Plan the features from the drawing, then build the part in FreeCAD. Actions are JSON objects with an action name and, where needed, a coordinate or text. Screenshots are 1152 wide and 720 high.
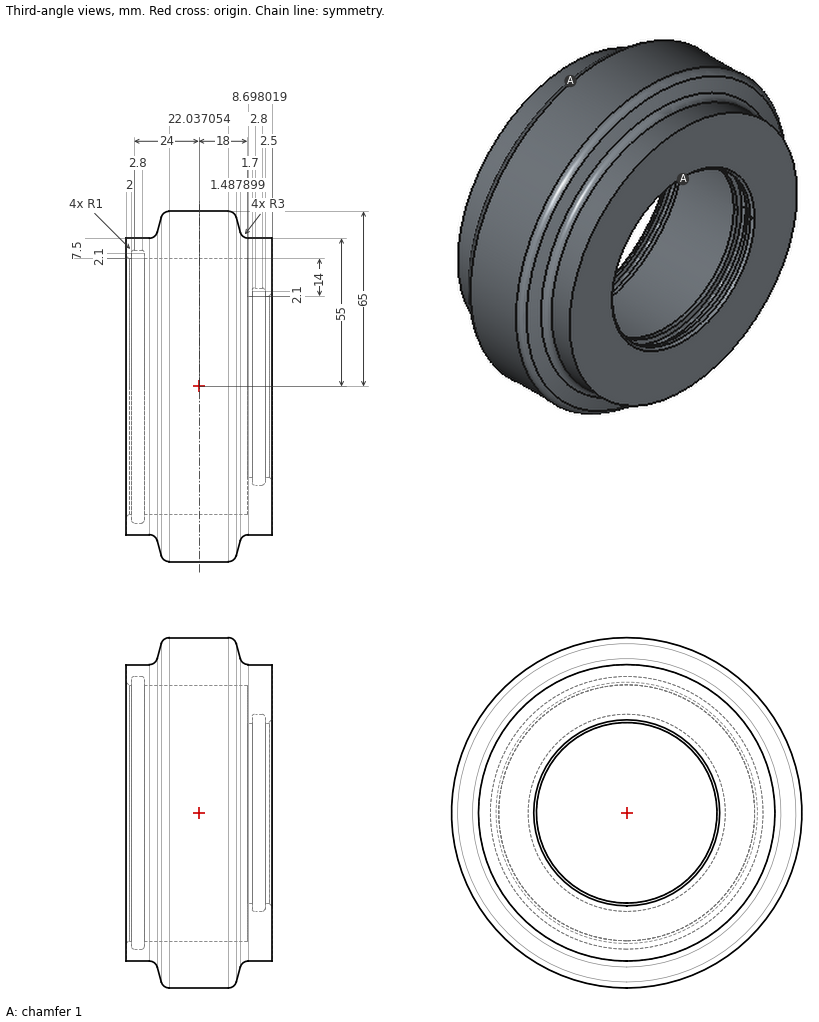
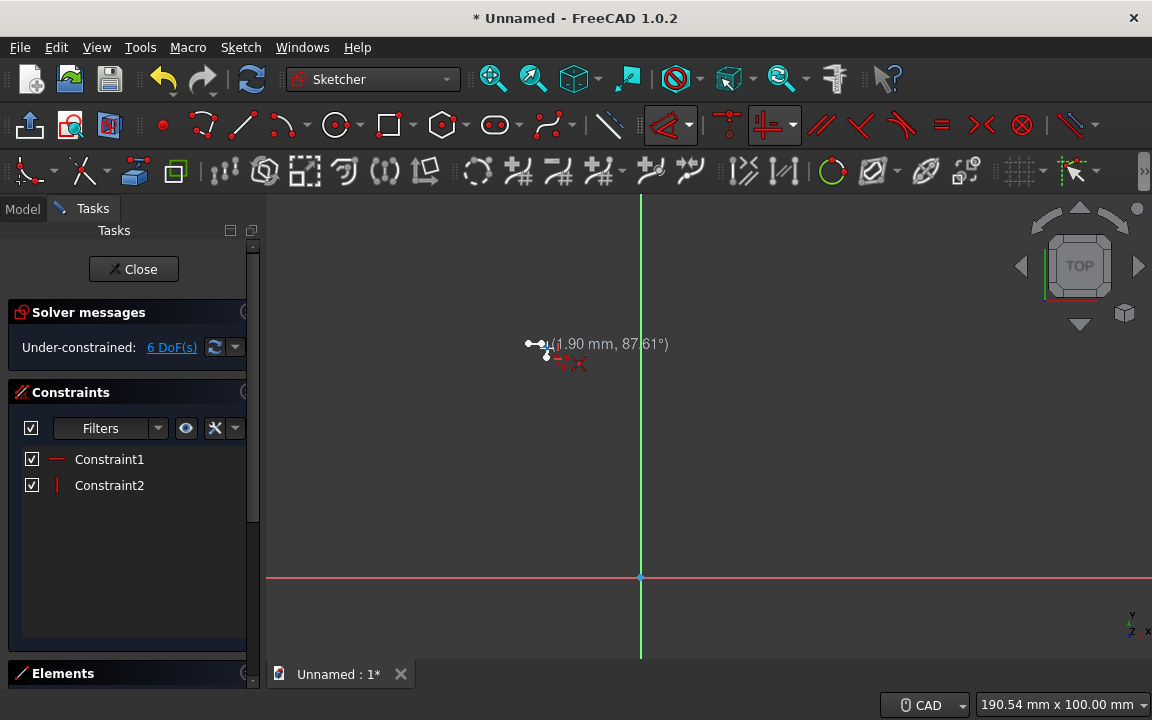
{"action": "left_click", "coordinate": [724, 357]}
{"action": "left_click", "coordinate": [724, 422]}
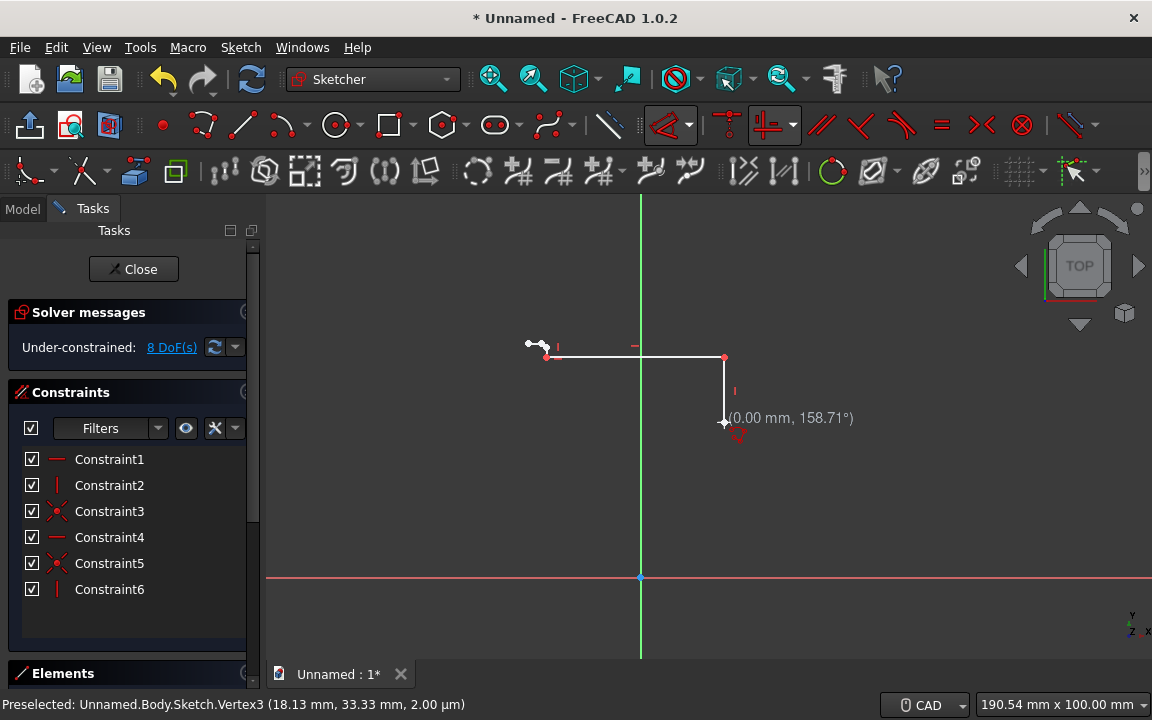
{"action": "scroll", "coordinate": [732, 422], "scroll_direction": "up", "scroll_amount": 4}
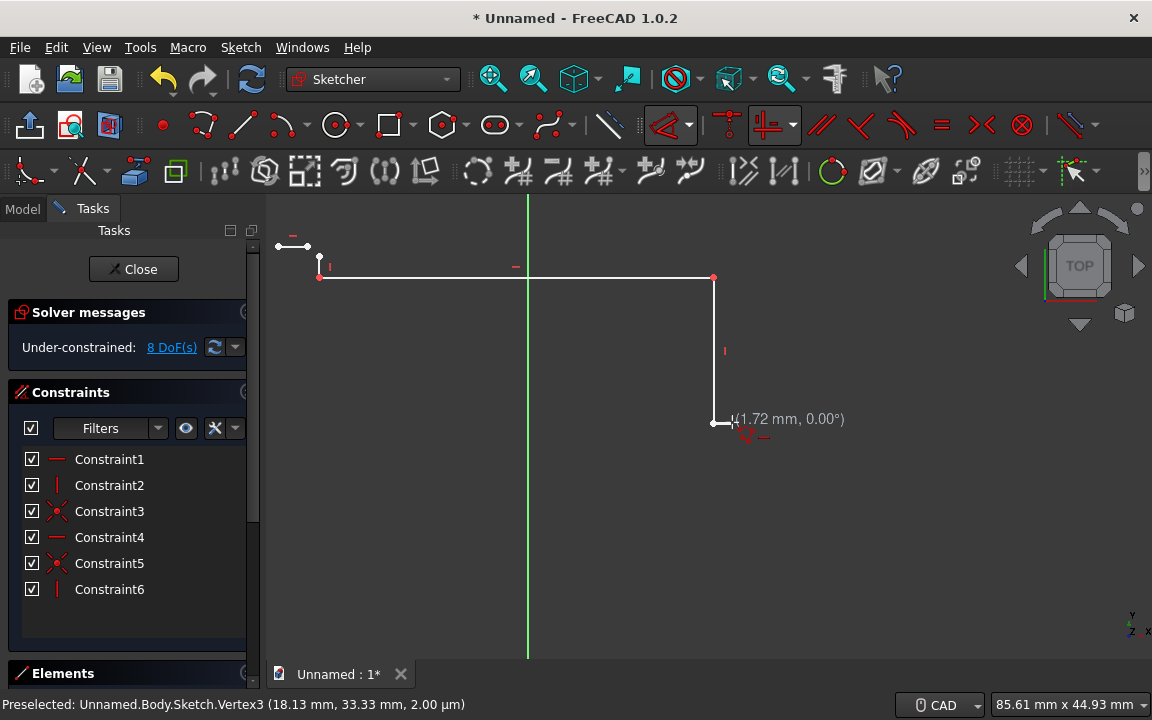
{"action": "left_click", "coordinate": [732, 421]}
{"action": "left_click", "coordinate": [732, 400]}
{"action": "right_click", "coordinate": [732, 400]}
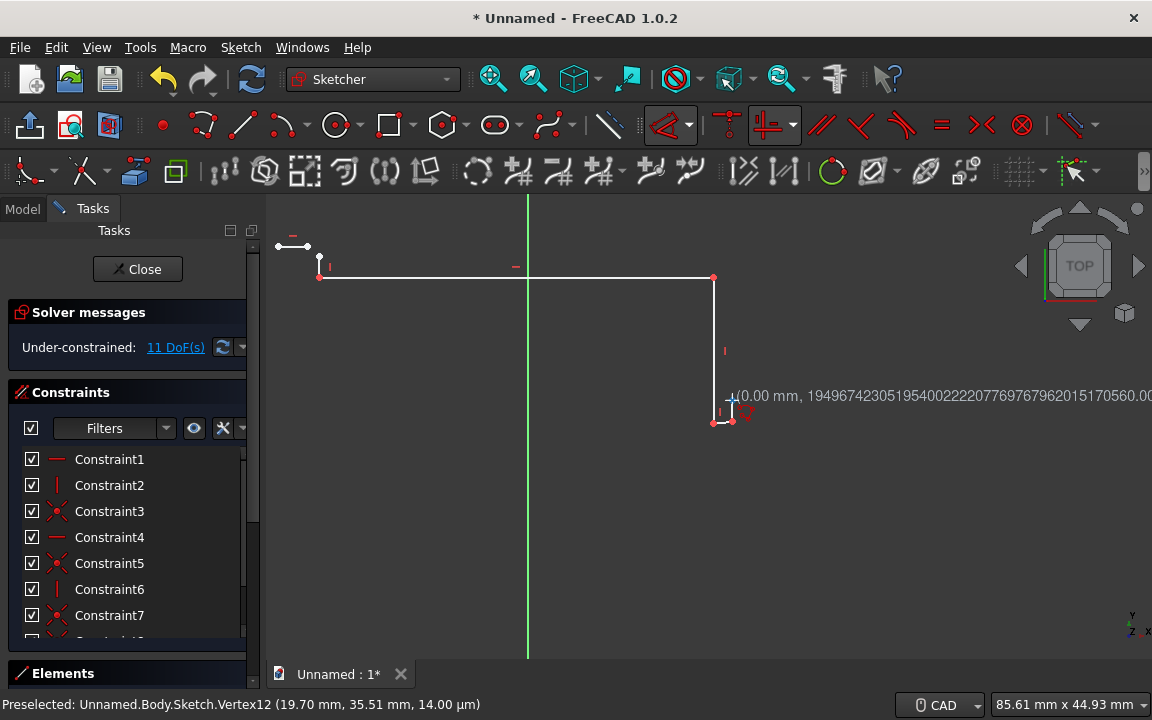
{"action": "key", "text": "g l"}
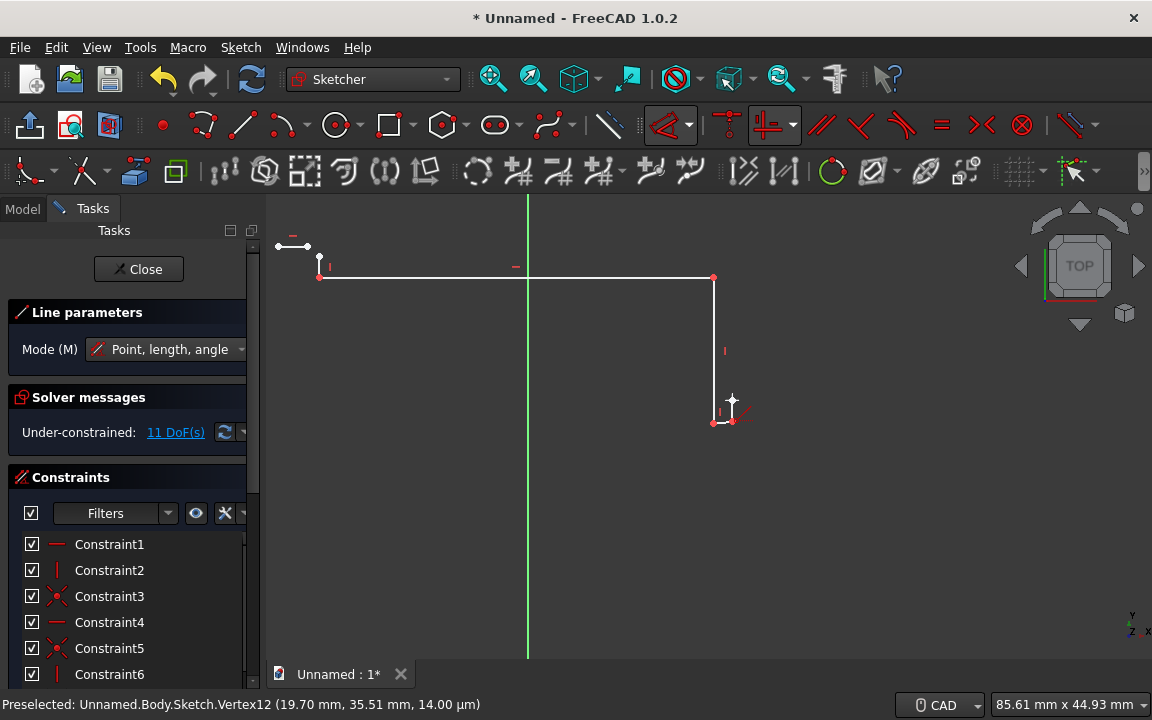
{"action": "left_click", "coordinate": [742, 390]}
{"action": "left_click", "coordinate": [771, 390]}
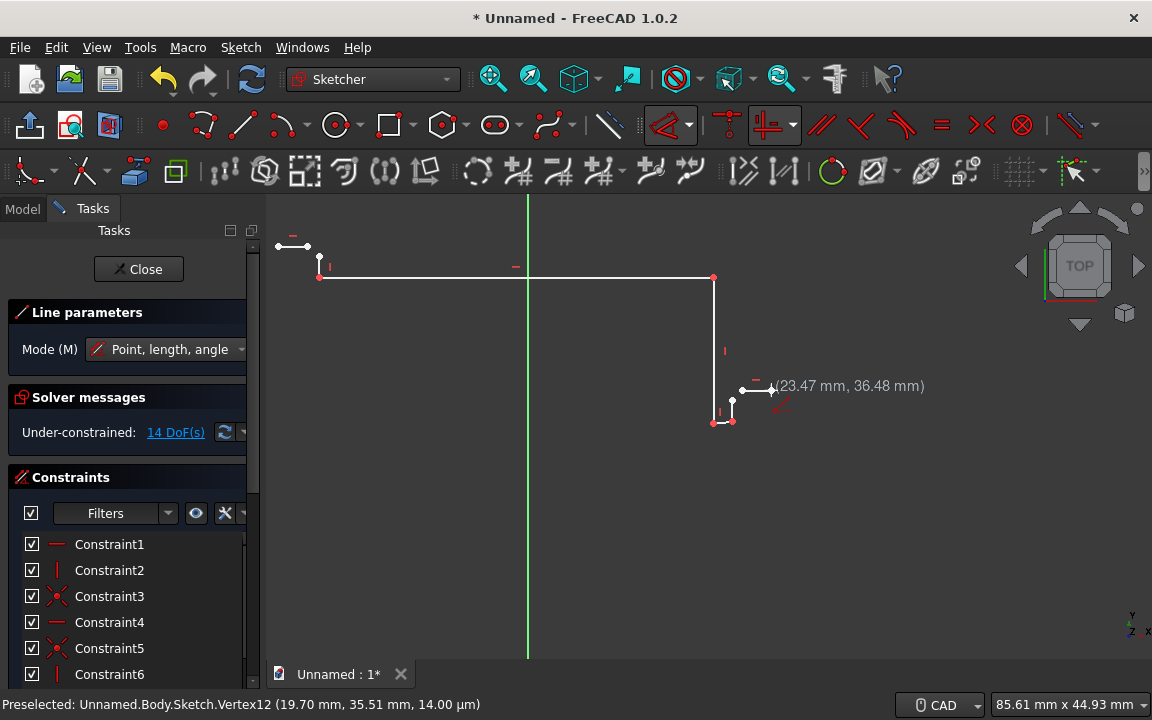
{"action": "left_click", "coordinate": [204, 126]}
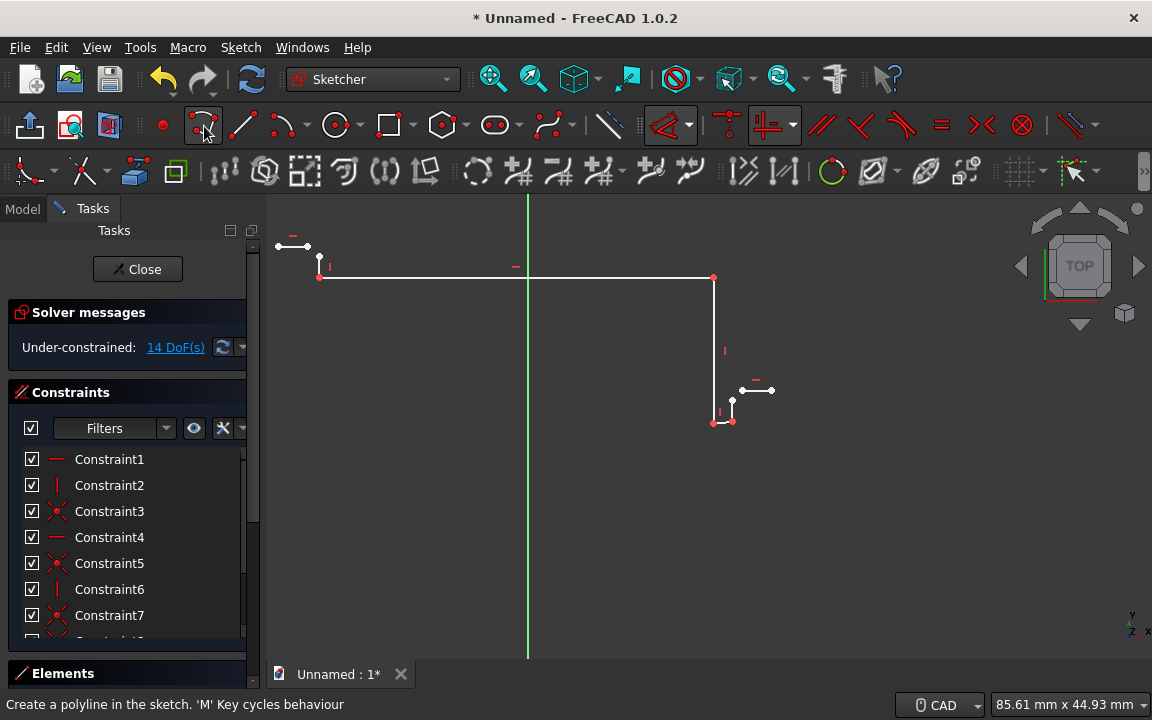
{"action": "left_click", "coordinate": [782, 400]}
{"action": "left_click", "coordinate": [782, 422]}
{"action": "left_click", "coordinate": [808, 422]}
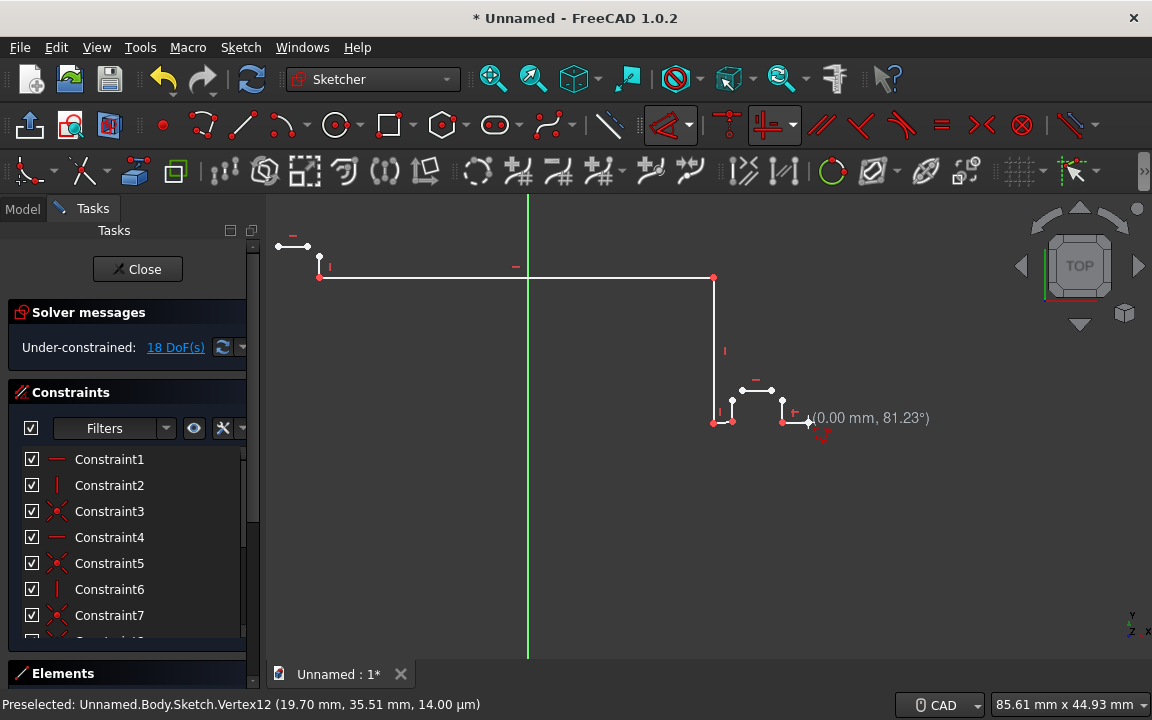
{"action": "scroll", "coordinate": [732, 422], "scroll_direction": "down", "scroll_amount": 4}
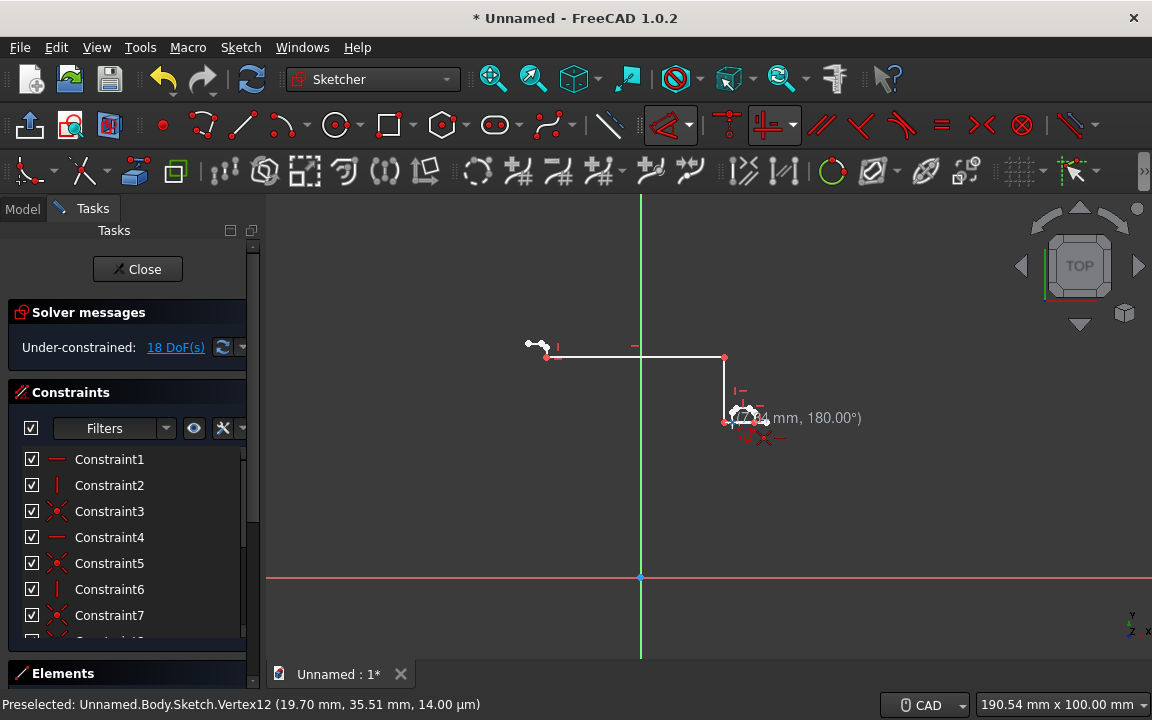
{"action": "left_click", "coordinate": [766, 322]}
{"action": "left_click", "coordinate": [726, 322]}
{"action": "right_click", "coordinate": [726, 322]}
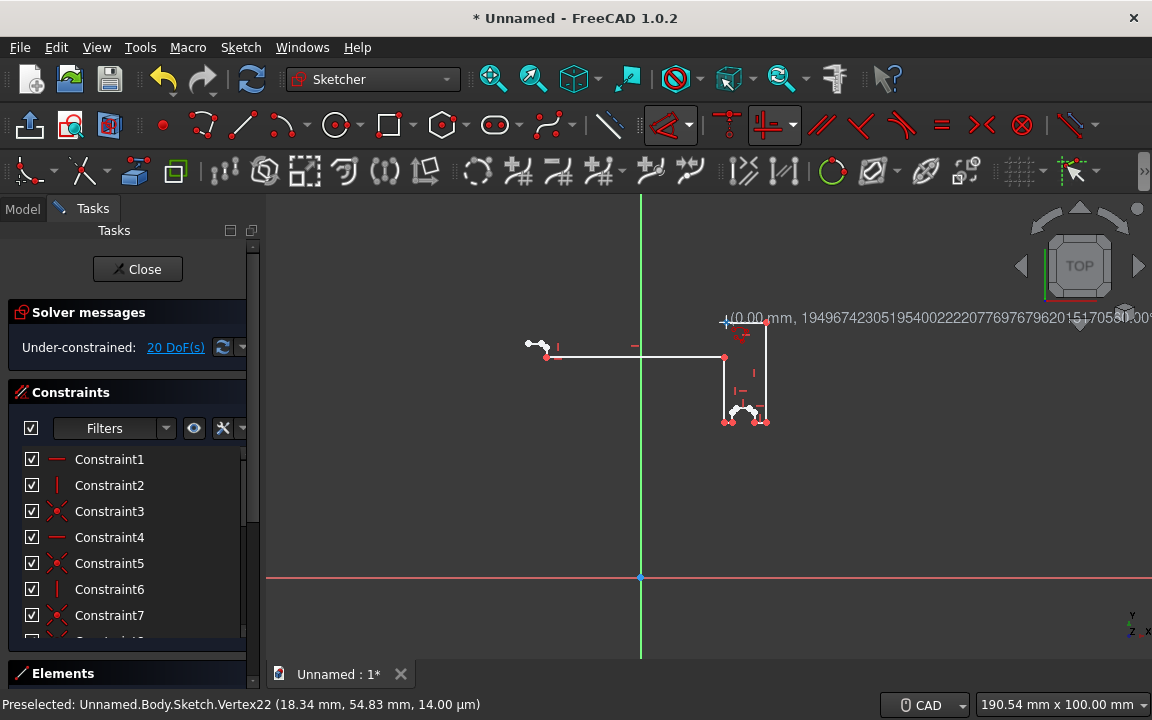
{"action": "left_click", "coordinate": [244, 126]}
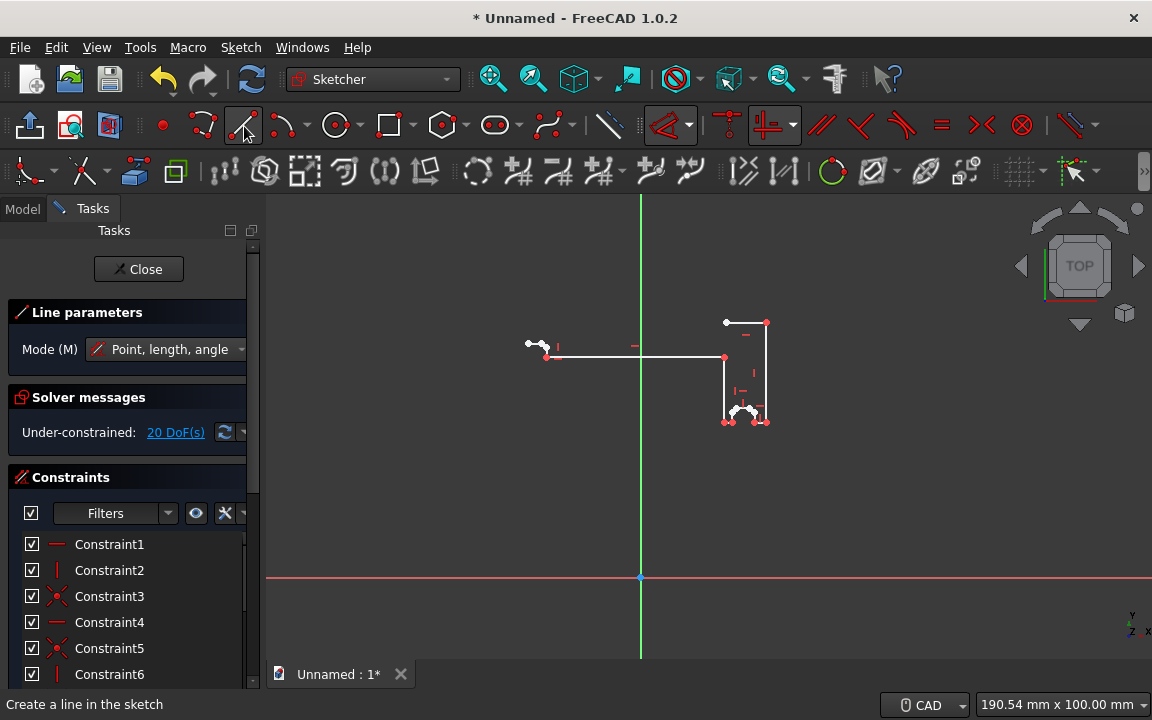
{"action": "left_click", "coordinate": [712, 312]}
{"action": "left_click", "coordinate": [705, 286]}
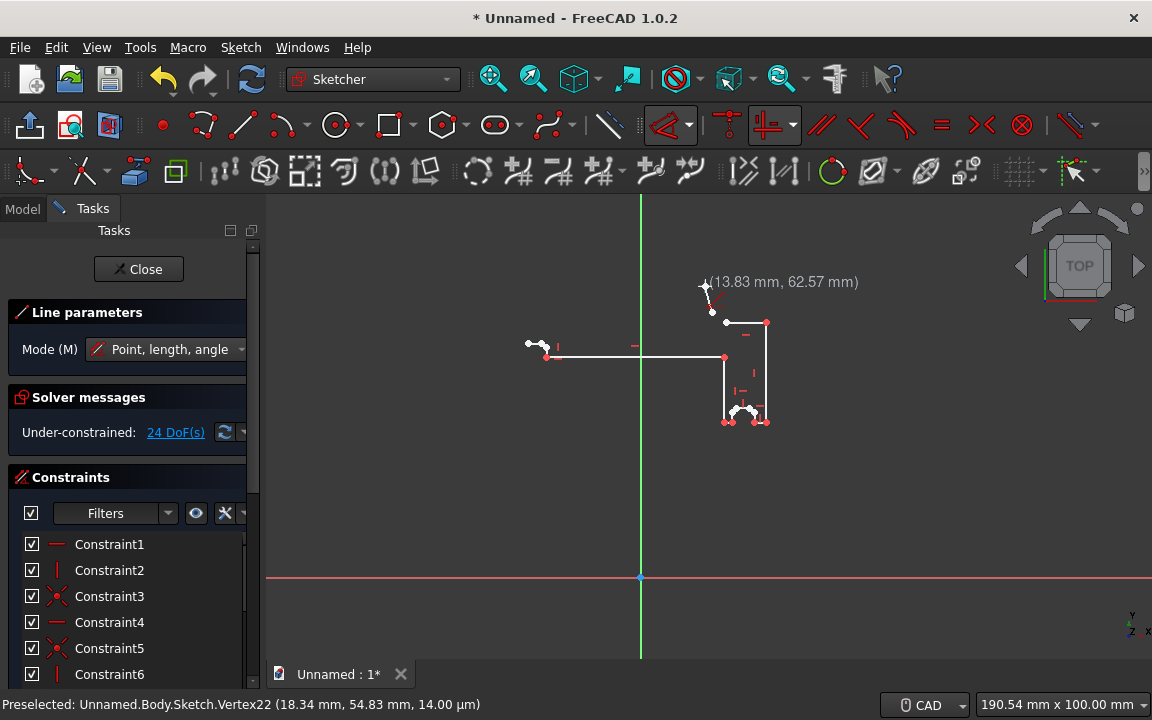
{"action": "left_click", "coordinate": [692, 276]}
{"action": "left_click", "coordinate": [589, 276]}